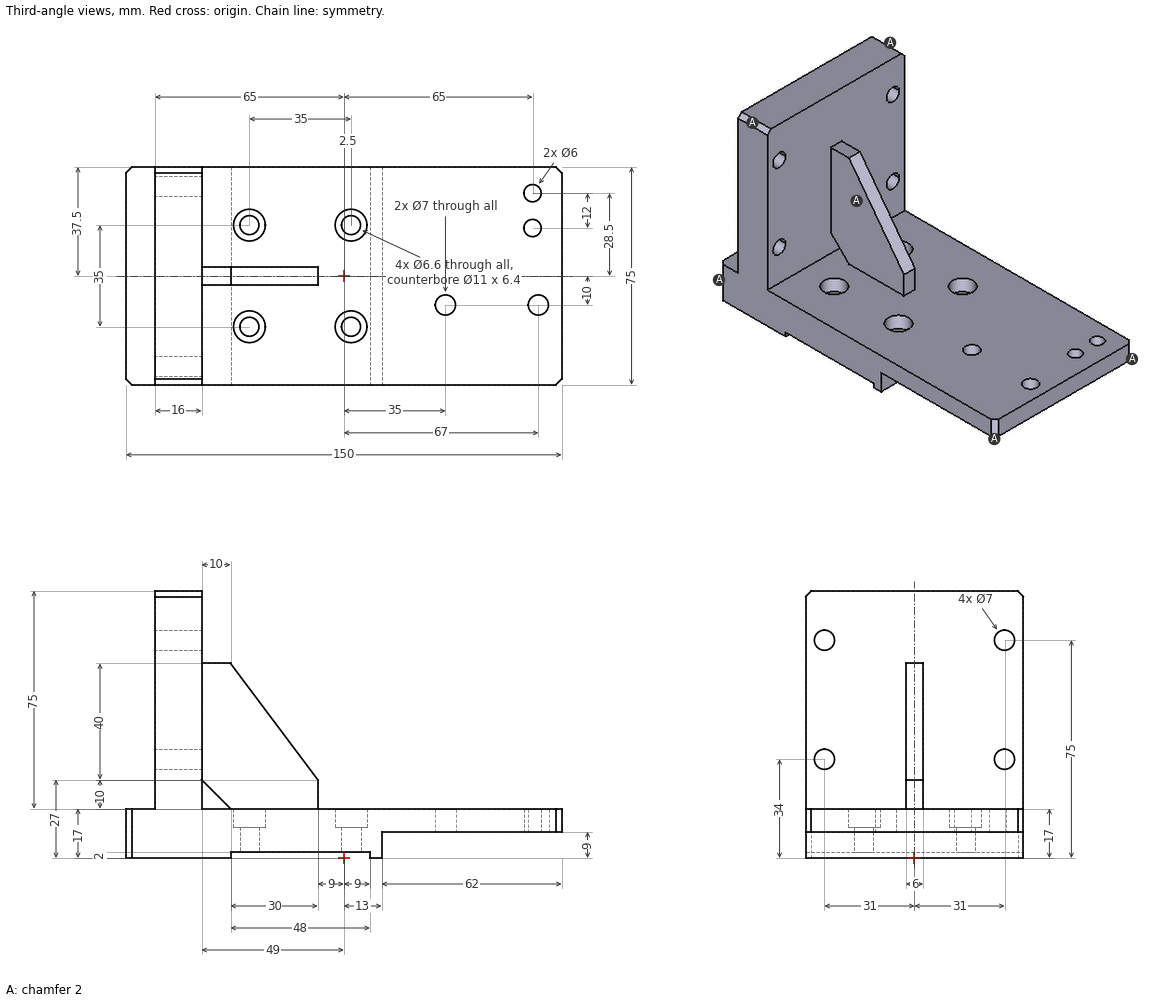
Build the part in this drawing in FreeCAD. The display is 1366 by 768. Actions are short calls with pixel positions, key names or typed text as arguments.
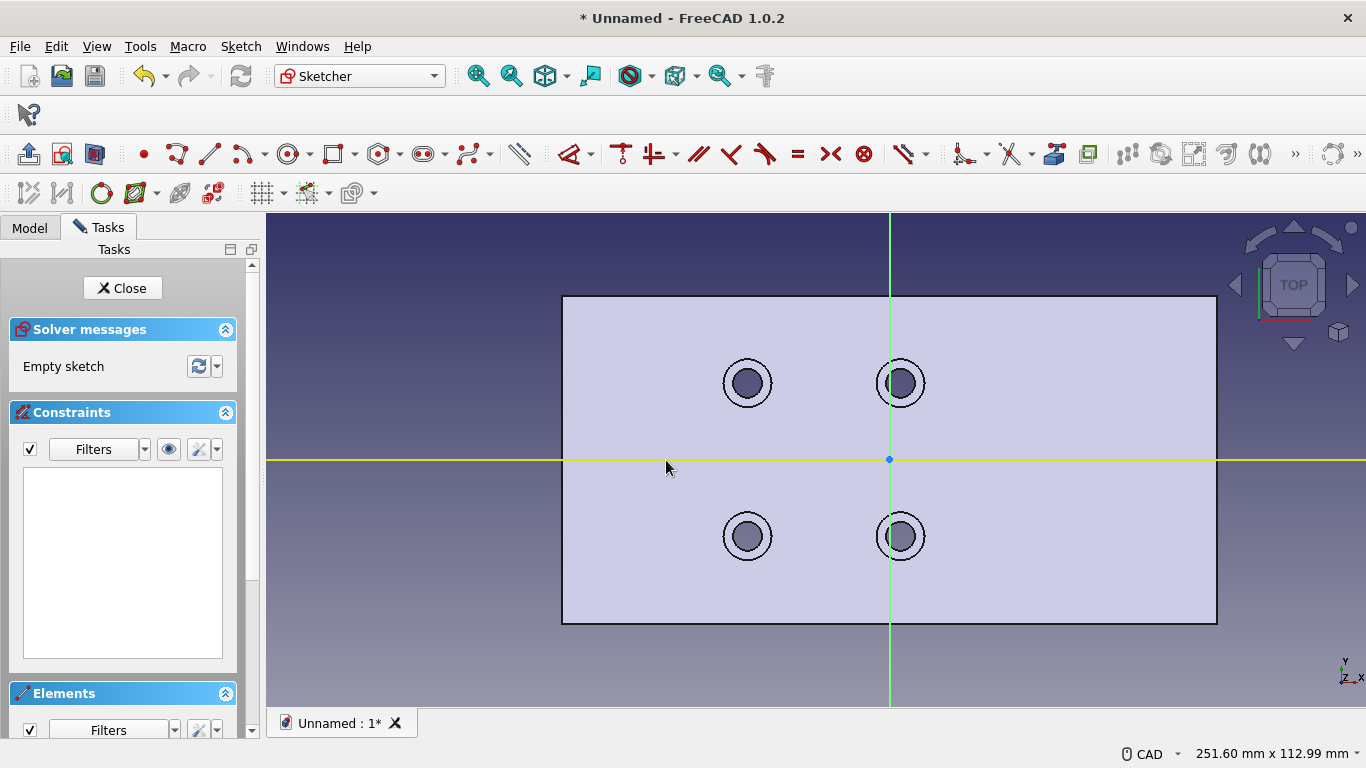
click(332, 154)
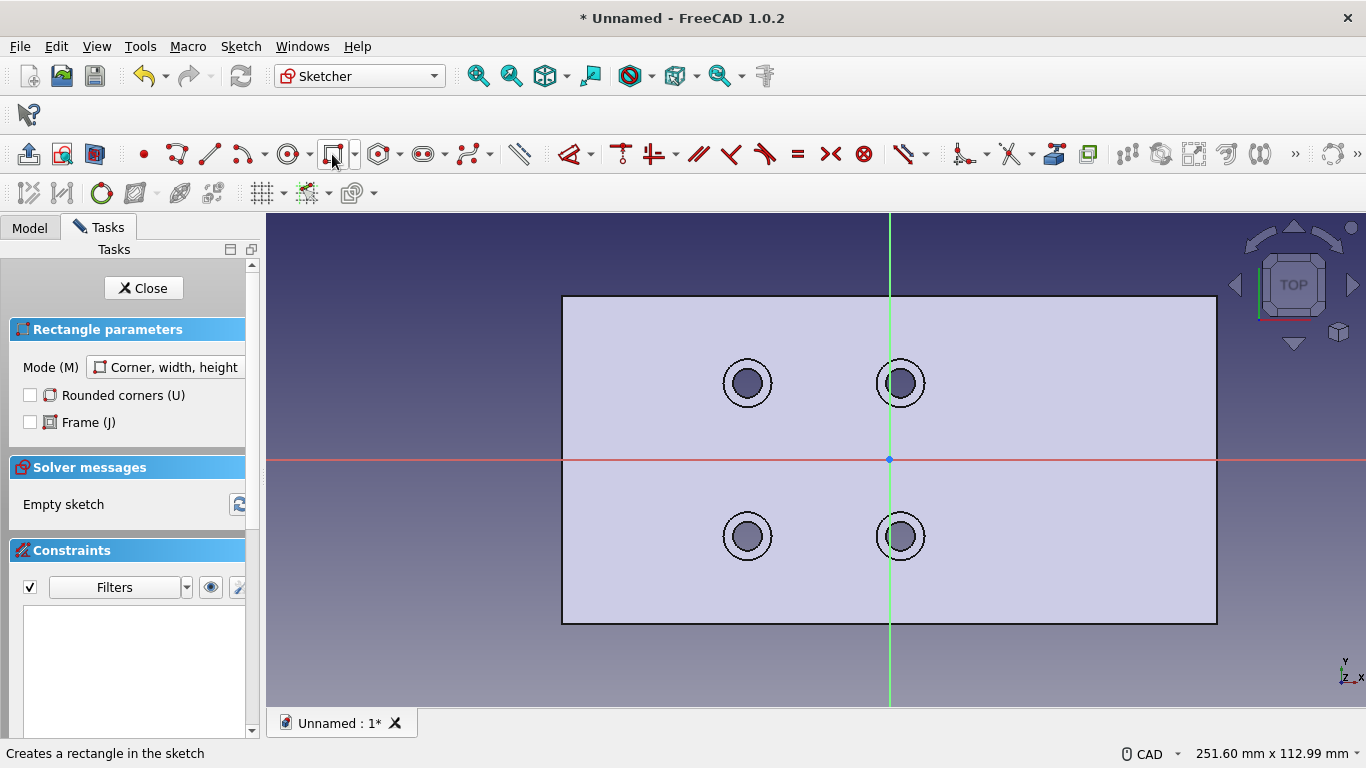
click(605, 296)
move(675, 624)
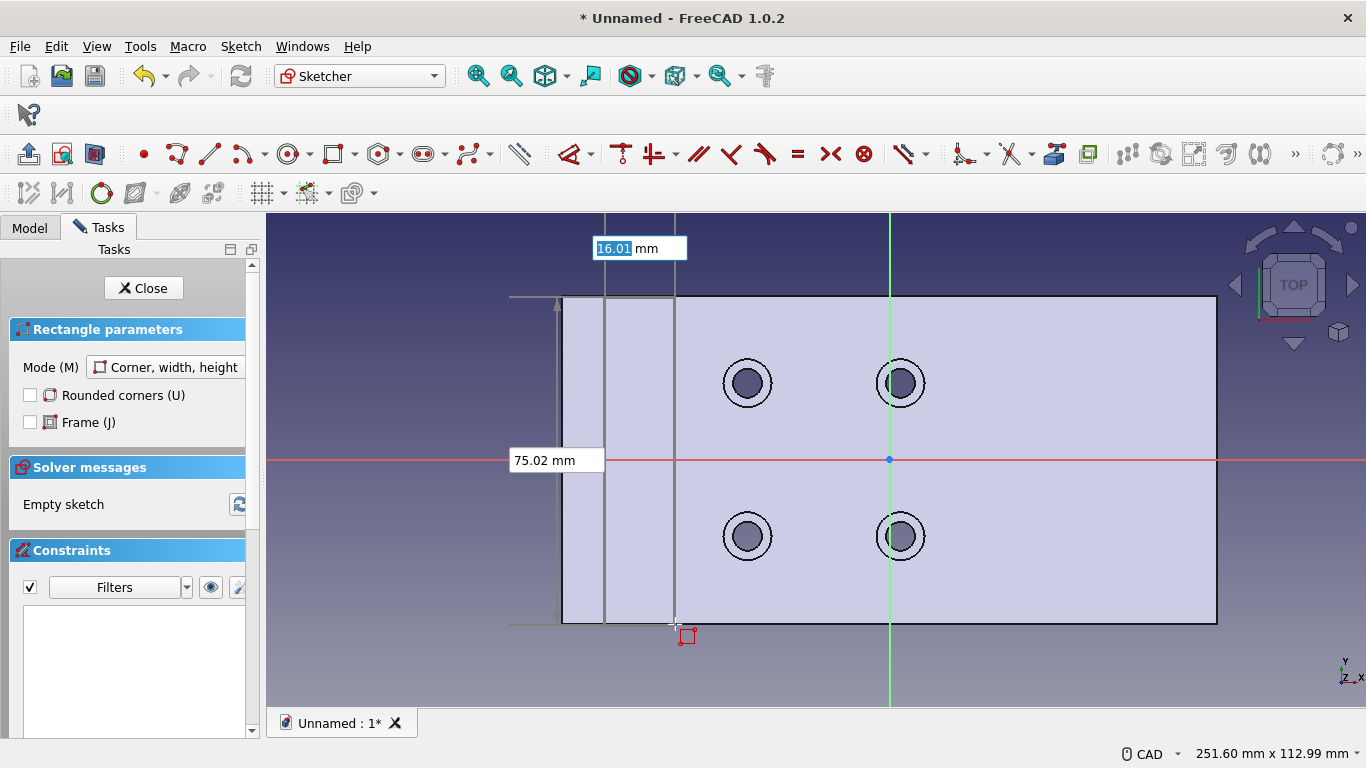
text(16)
key(Tab)
text(75)
key(Return)
key(Escape)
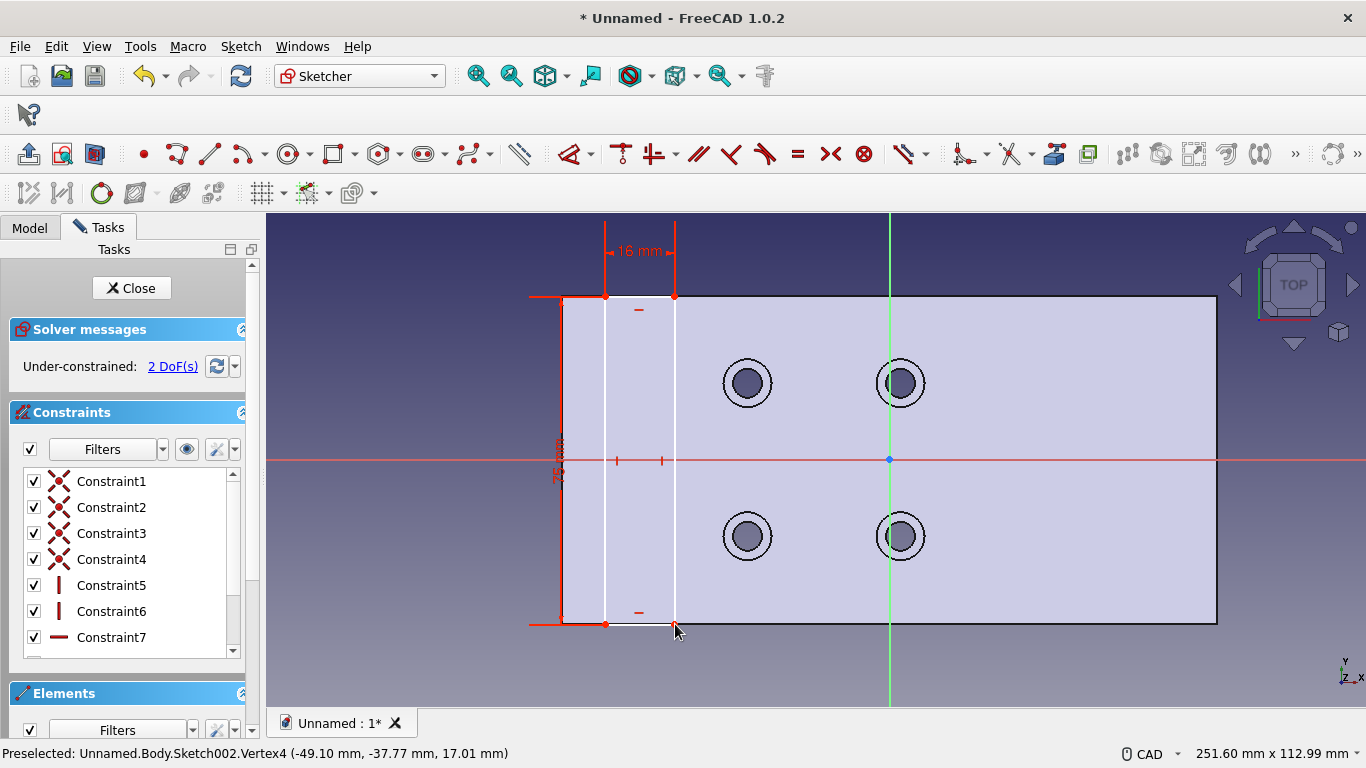
click(568, 154)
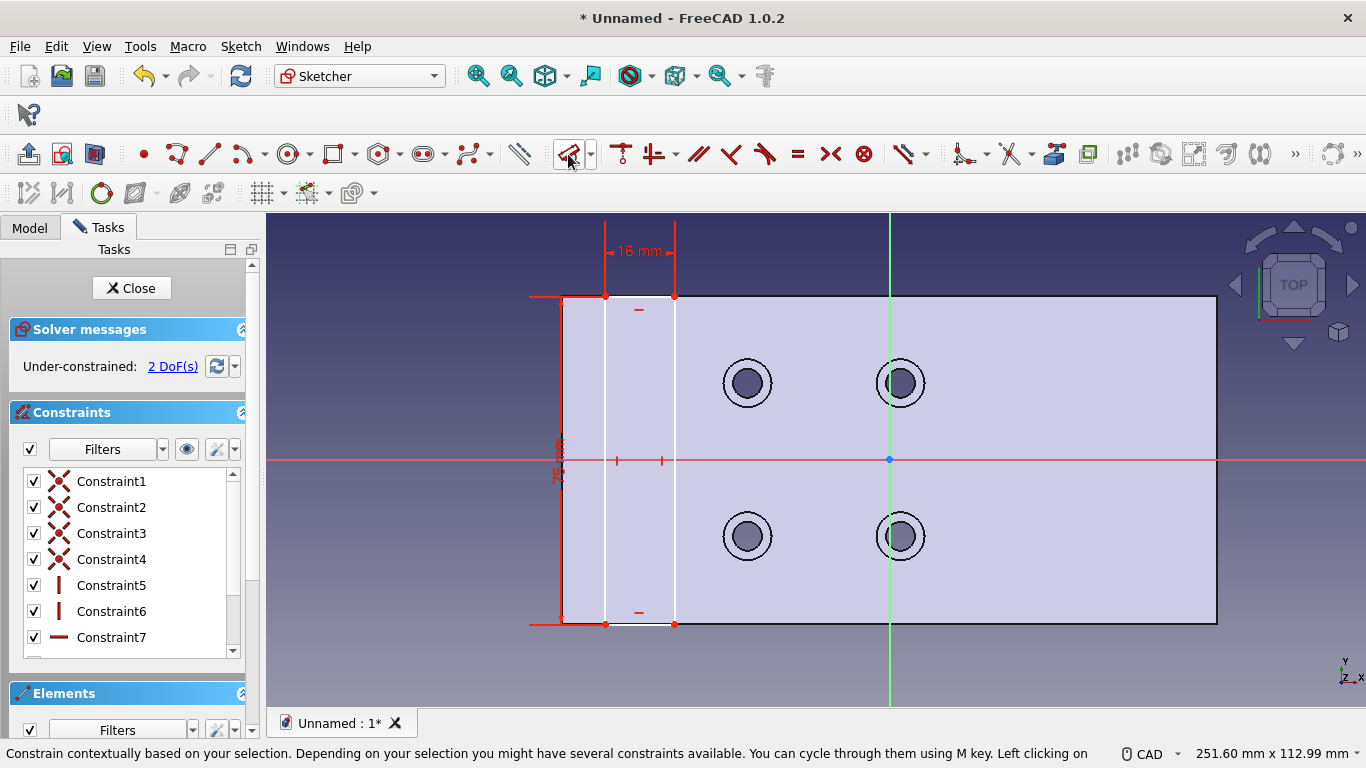
click(605, 297)
click(747, 263)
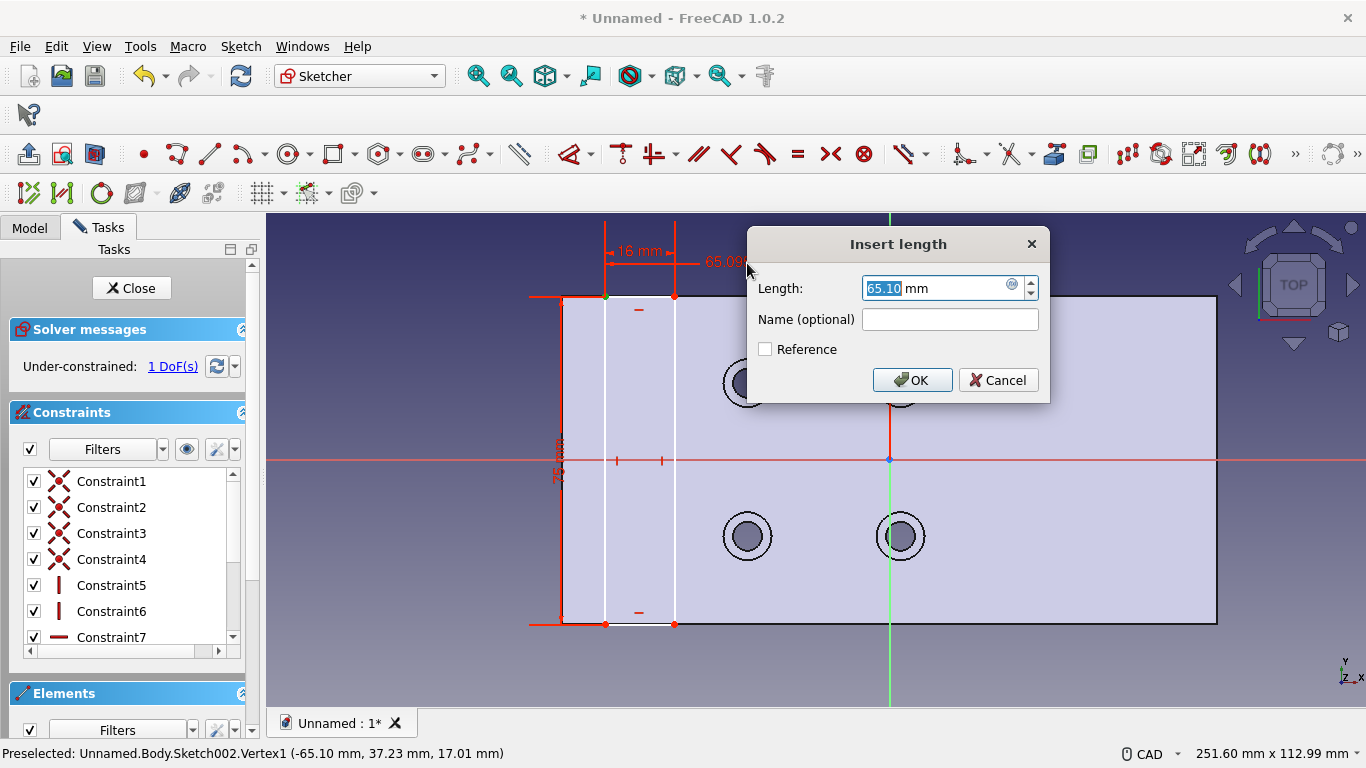
text(65)
key(Return)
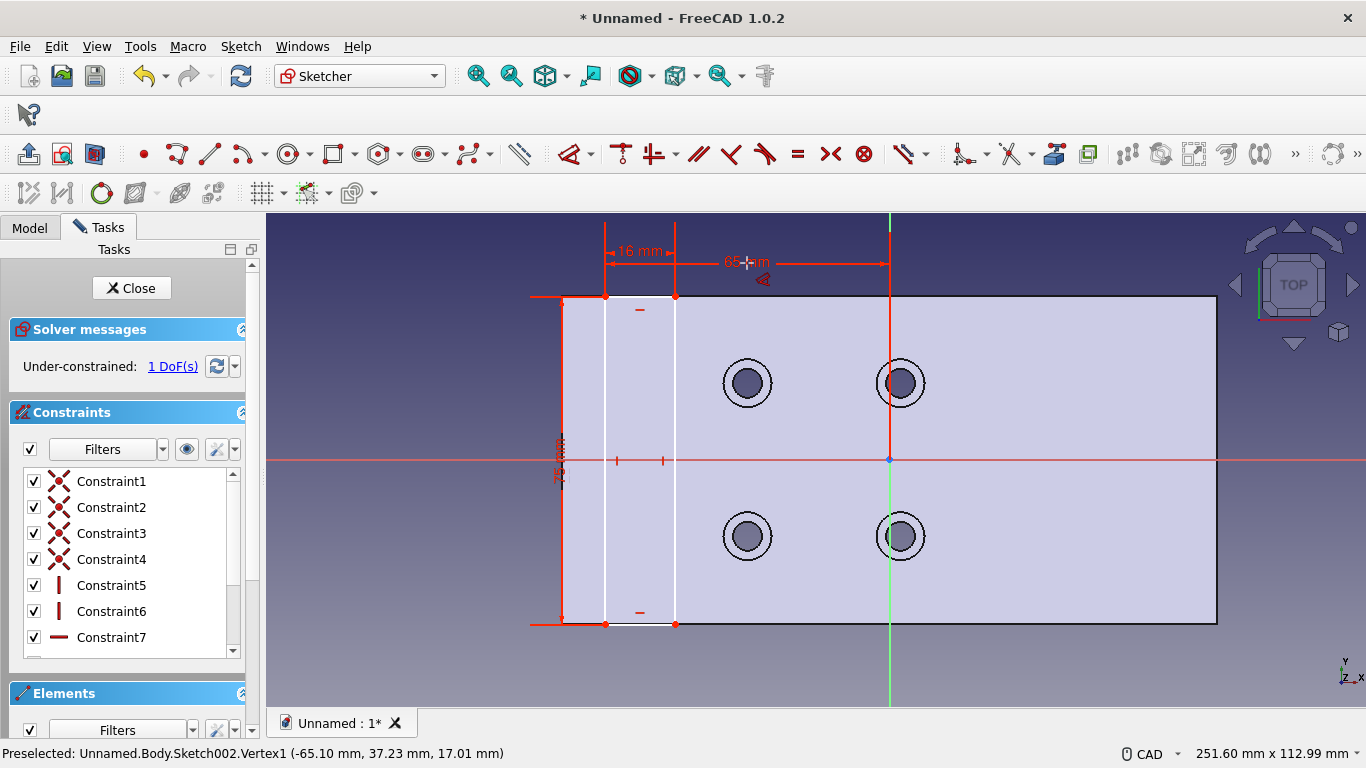
click(605, 297)
click(924, 378)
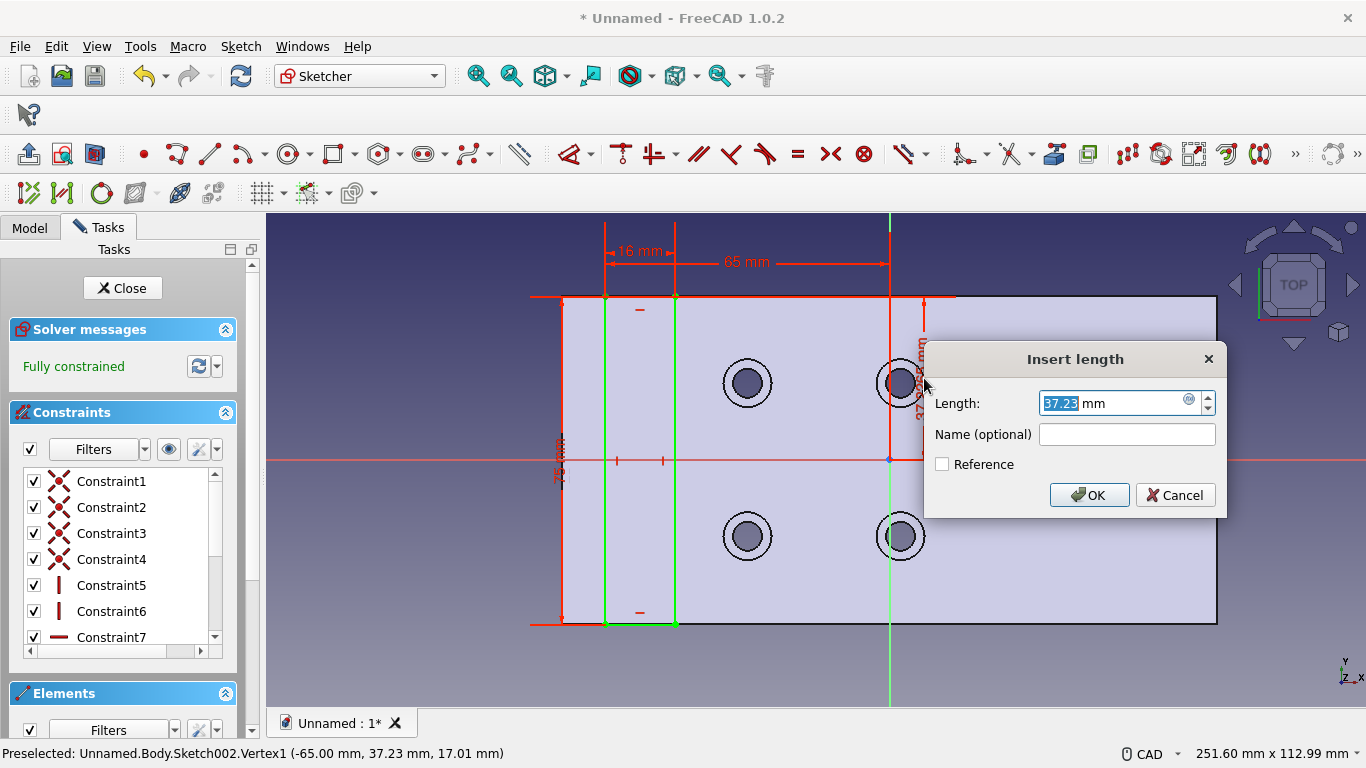
text(37.5)
key(Return)
key(Escape)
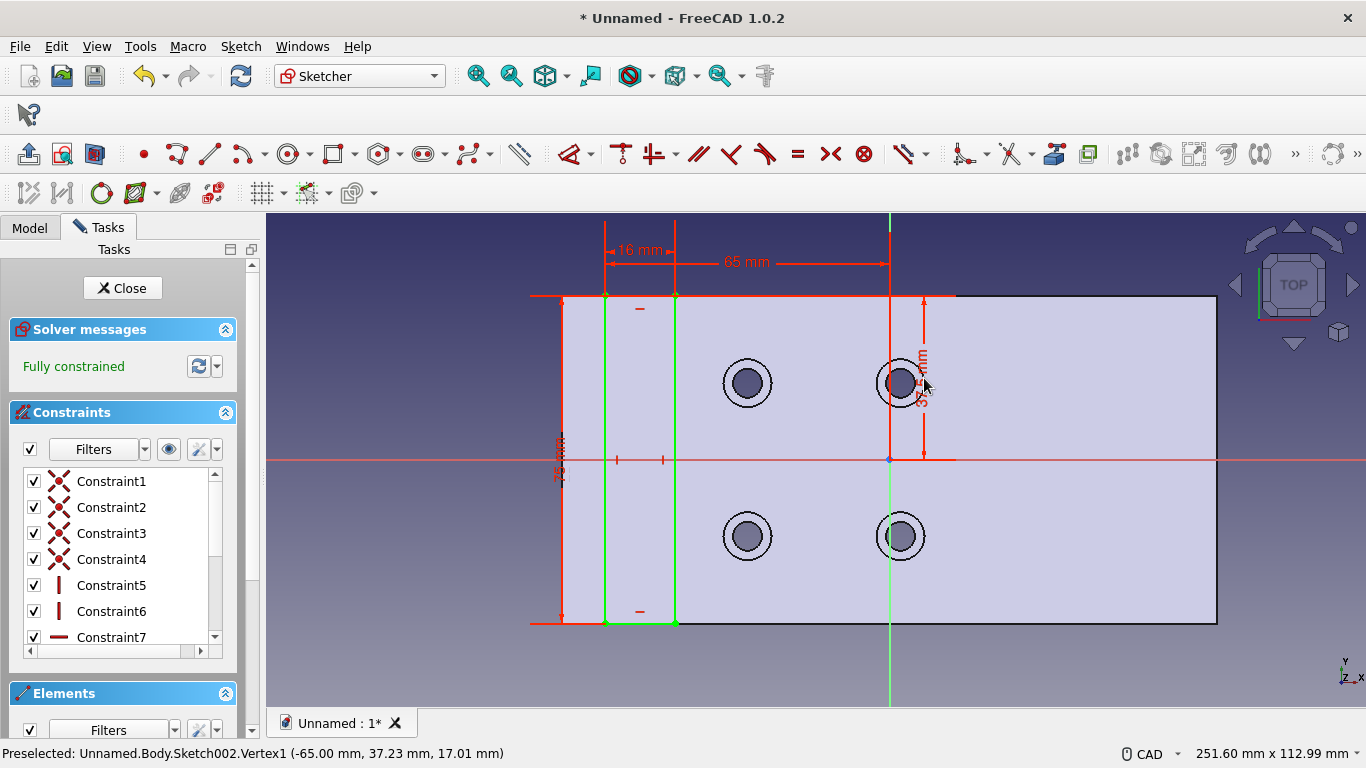
click(123, 288)